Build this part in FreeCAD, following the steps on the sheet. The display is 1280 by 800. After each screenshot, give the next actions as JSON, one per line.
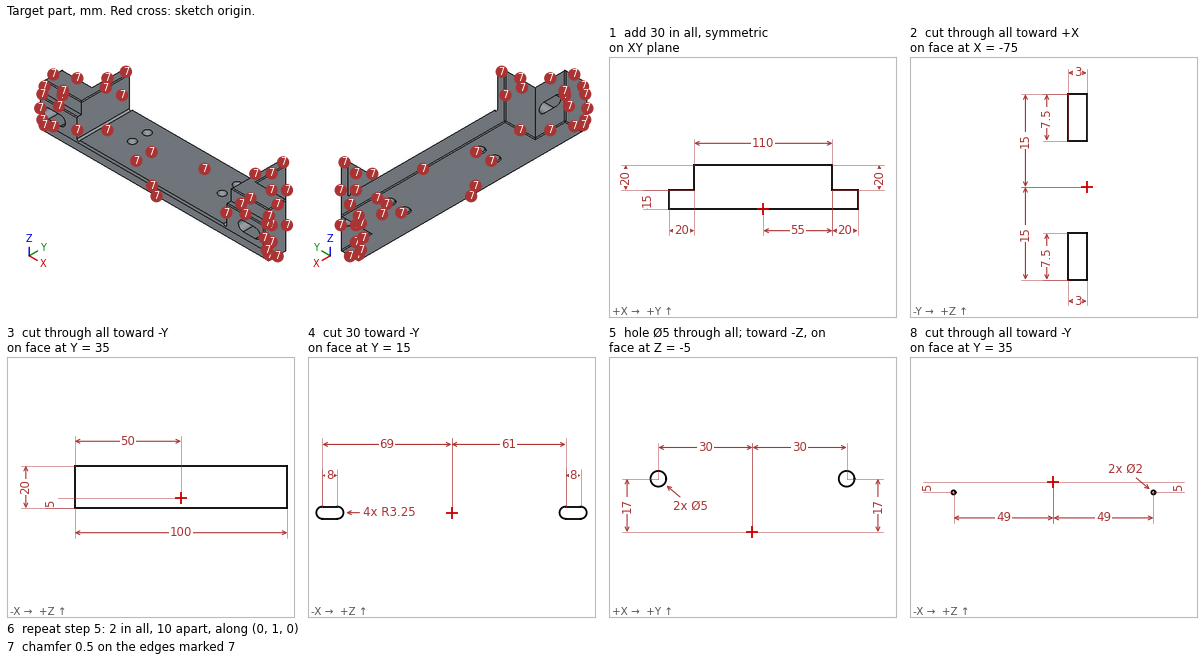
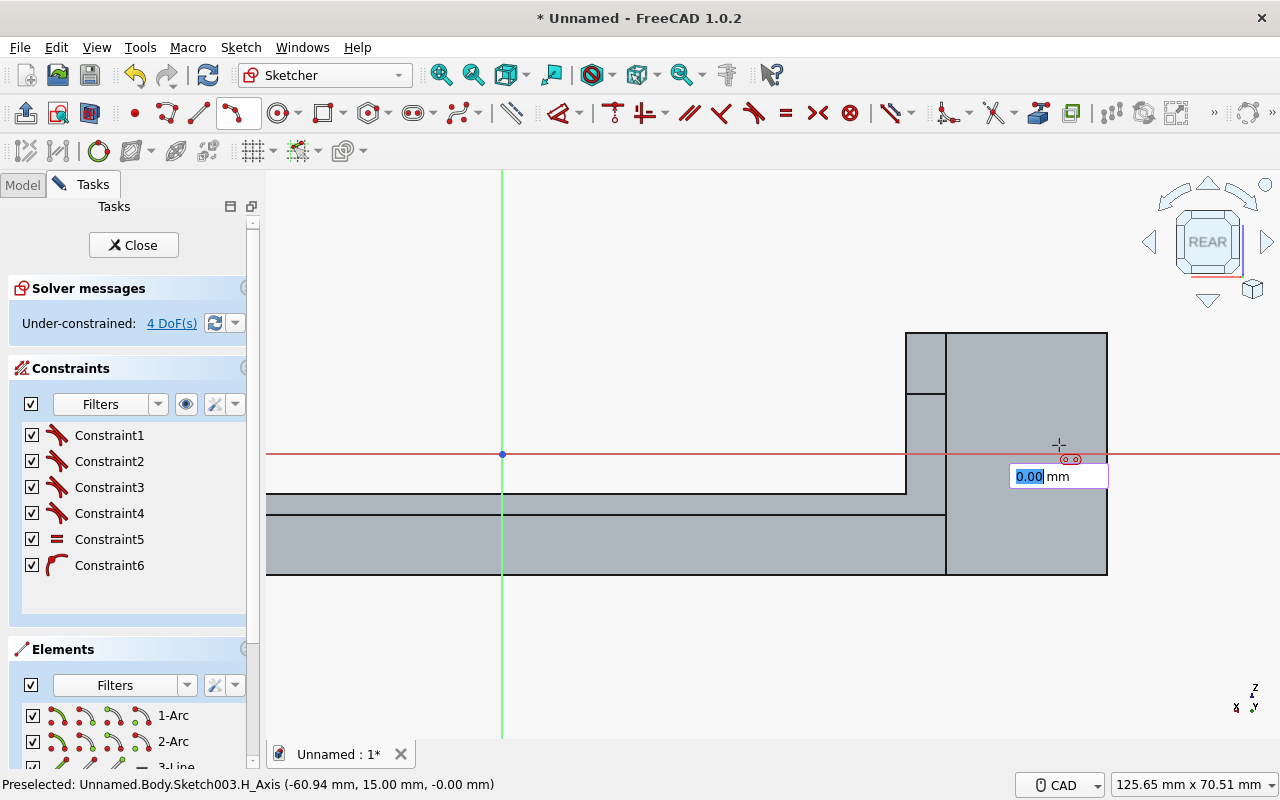
{"action": "left_click", "coordinate": [1027, 480]}
{"action": "key", "text": "Escape"}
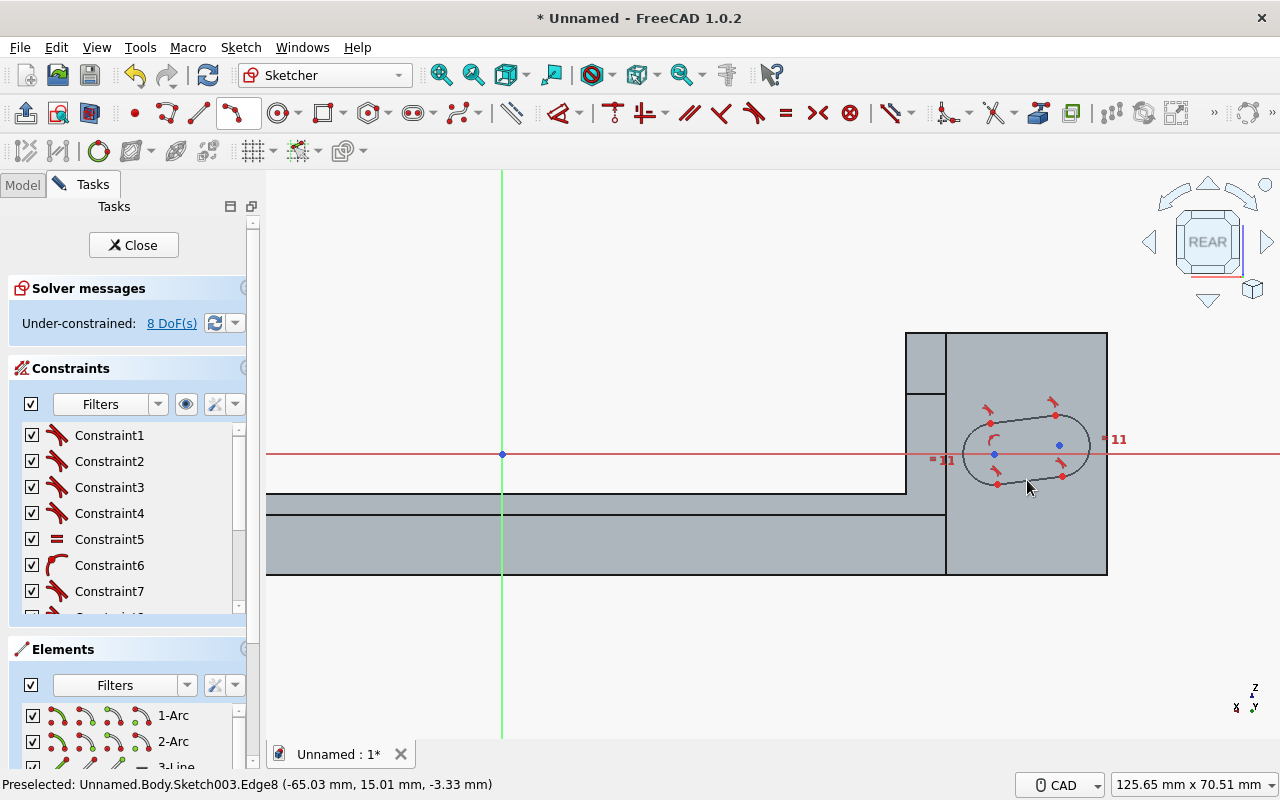
{"action": "scroll", "coordinate": [951, 455], "scroll_direction": "down", "scroll_amount": 3}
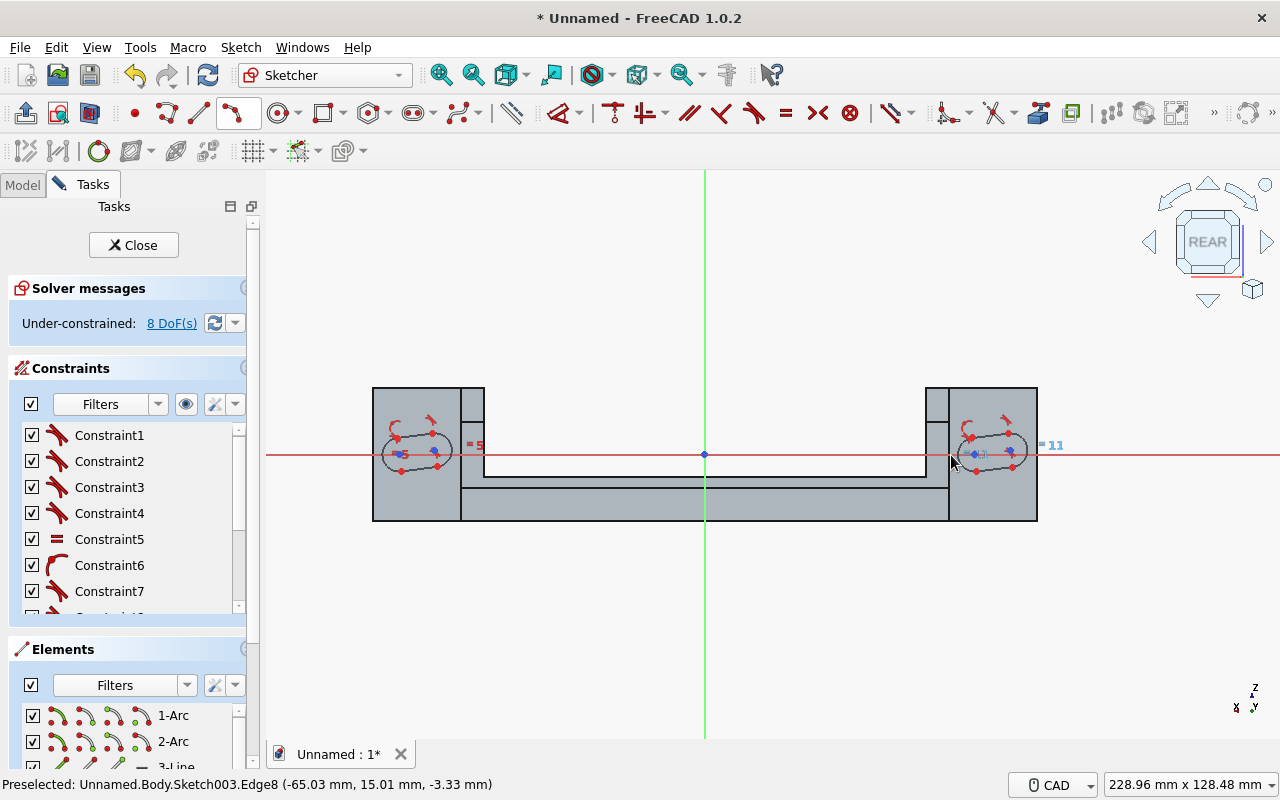
{"action": "scroll", "coordinate": [408, 437], "scroll_direction": "up", "scroll_amount": 2}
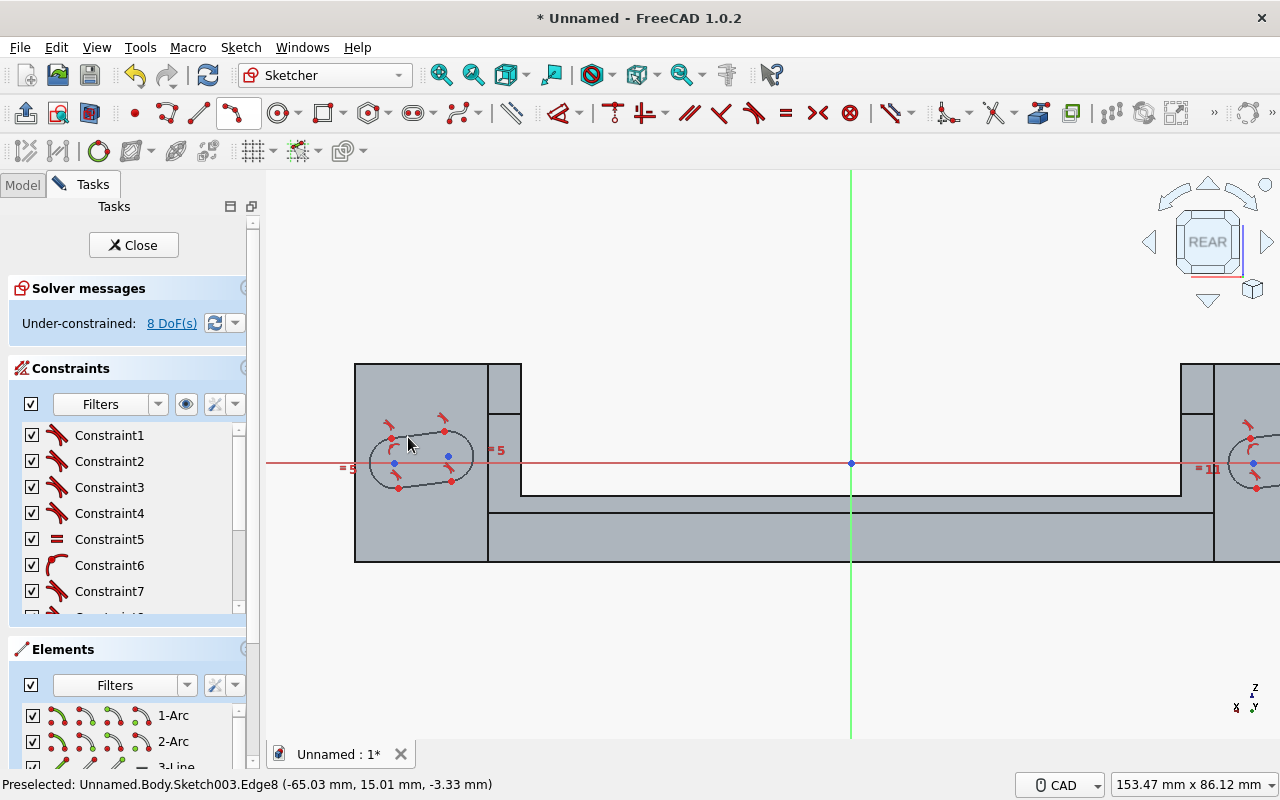
{"action": "left_click", "coordinate": [408, 436]}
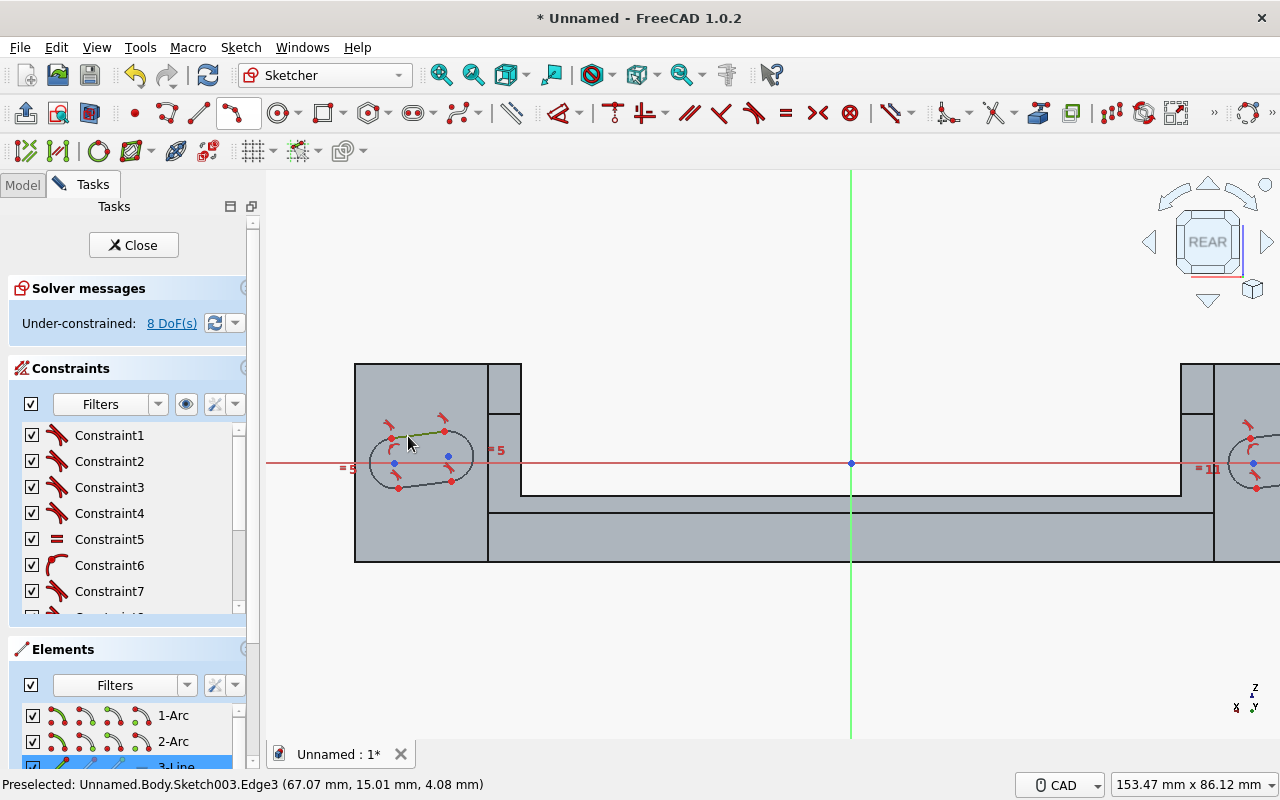
{"action": "key", "text": "h"}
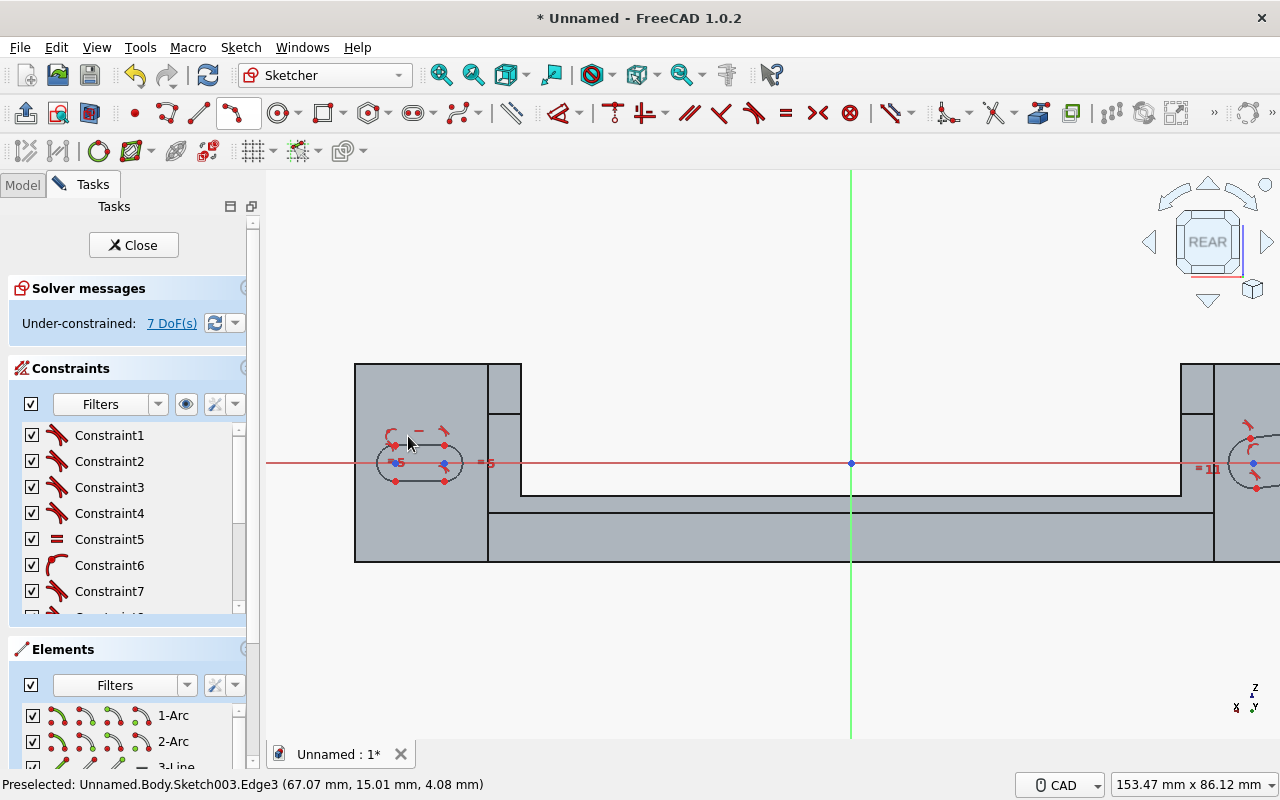
{"action": "scroll", "coordinate": [407, 437], "scroll_direction": "down", "scroll_amount": 2}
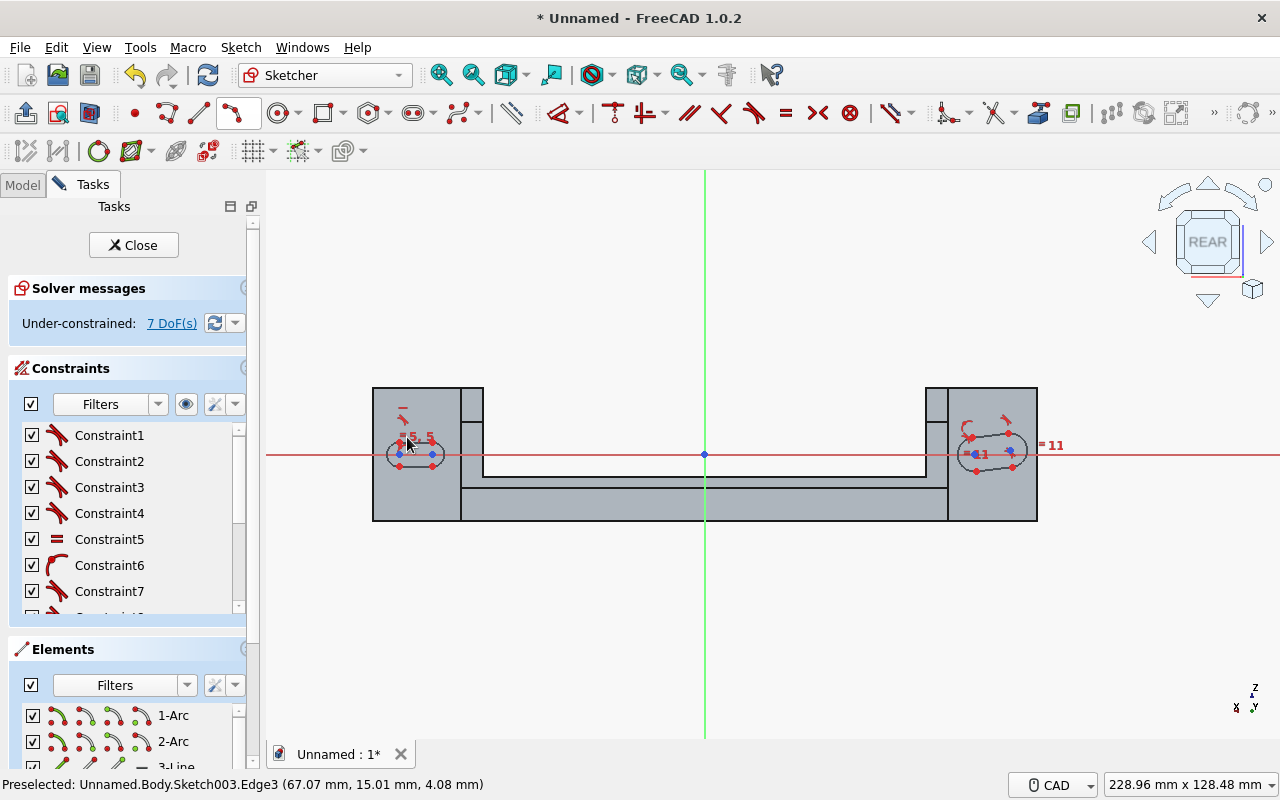
{"action": "scroll", "coordinate": [983, 437], "scroll_direction": "up", "scroll_amount": 2}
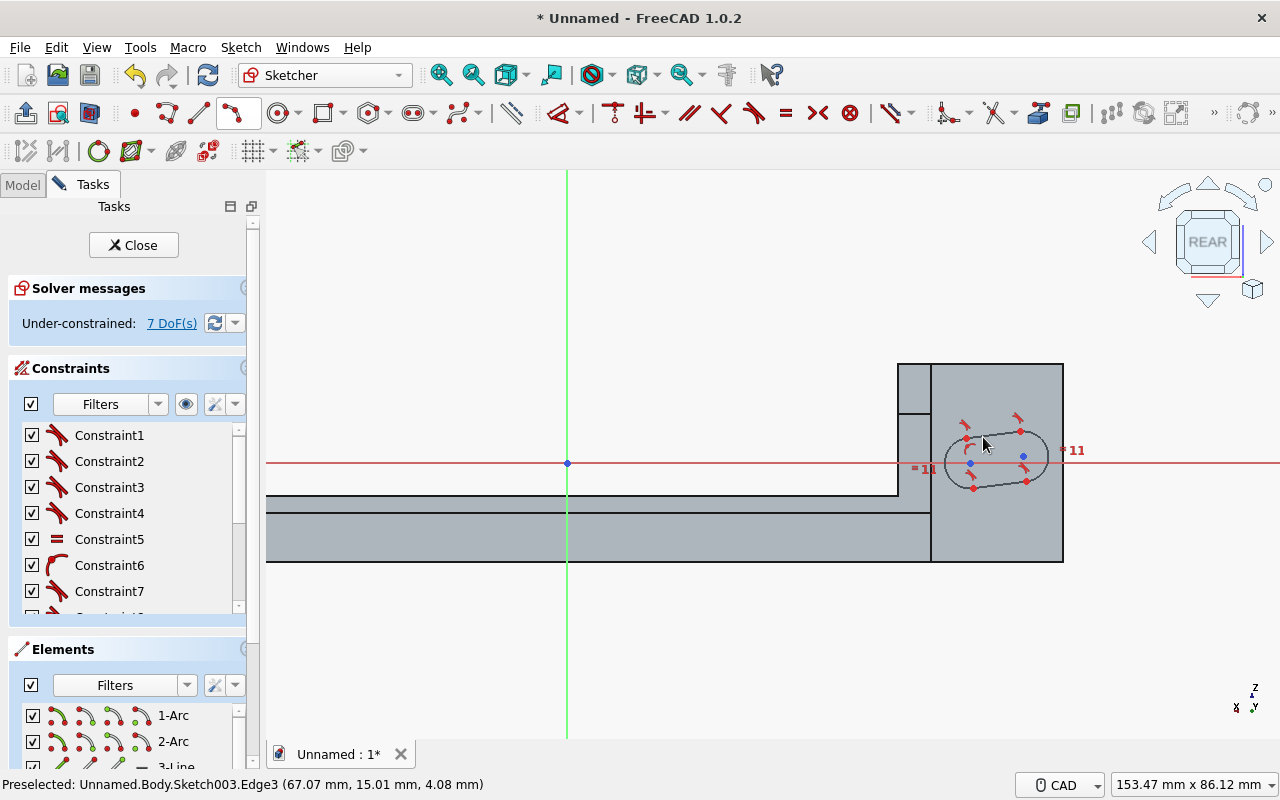
{"action": "left_click", "coordinate": [983, 436]}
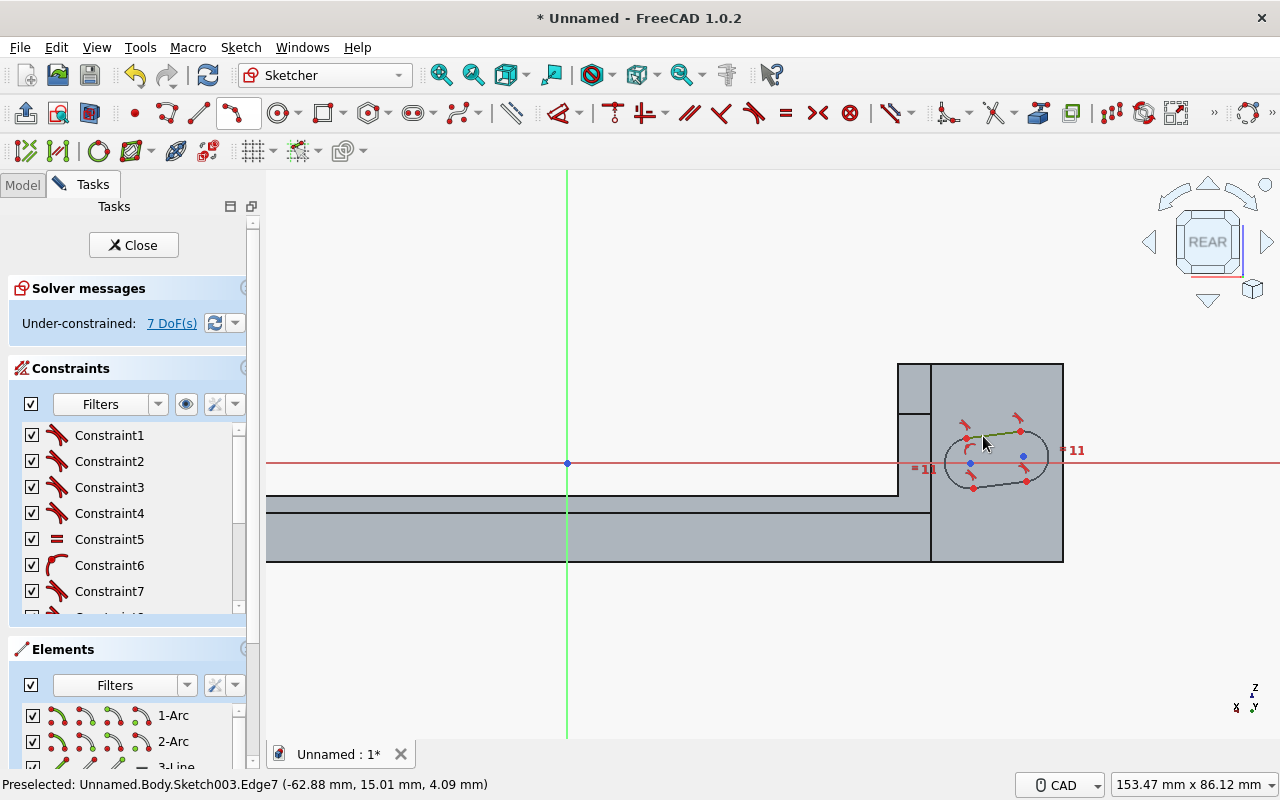
{"action": "key", "text": "h"}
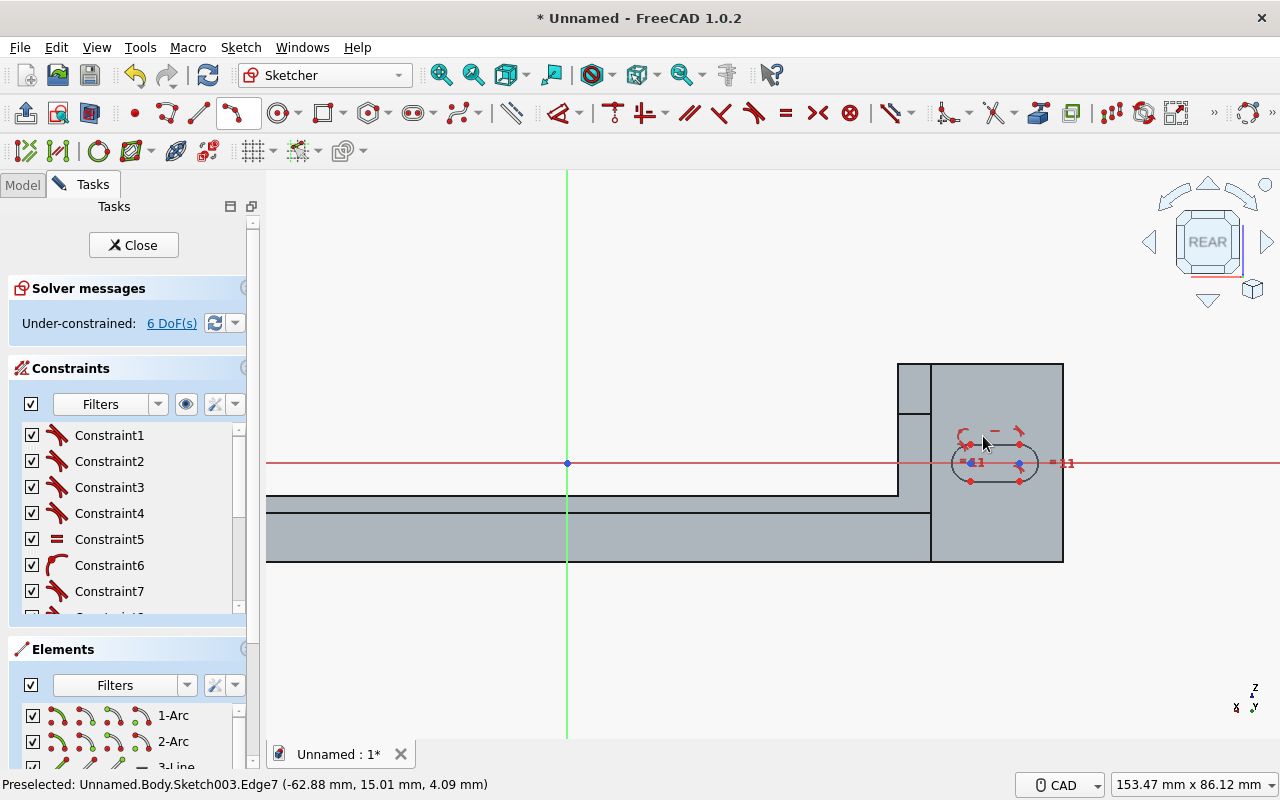
{"action": "scroll", "coordinate": [983, 437], "scroll_direction": "down", "scroll_amount": 2}